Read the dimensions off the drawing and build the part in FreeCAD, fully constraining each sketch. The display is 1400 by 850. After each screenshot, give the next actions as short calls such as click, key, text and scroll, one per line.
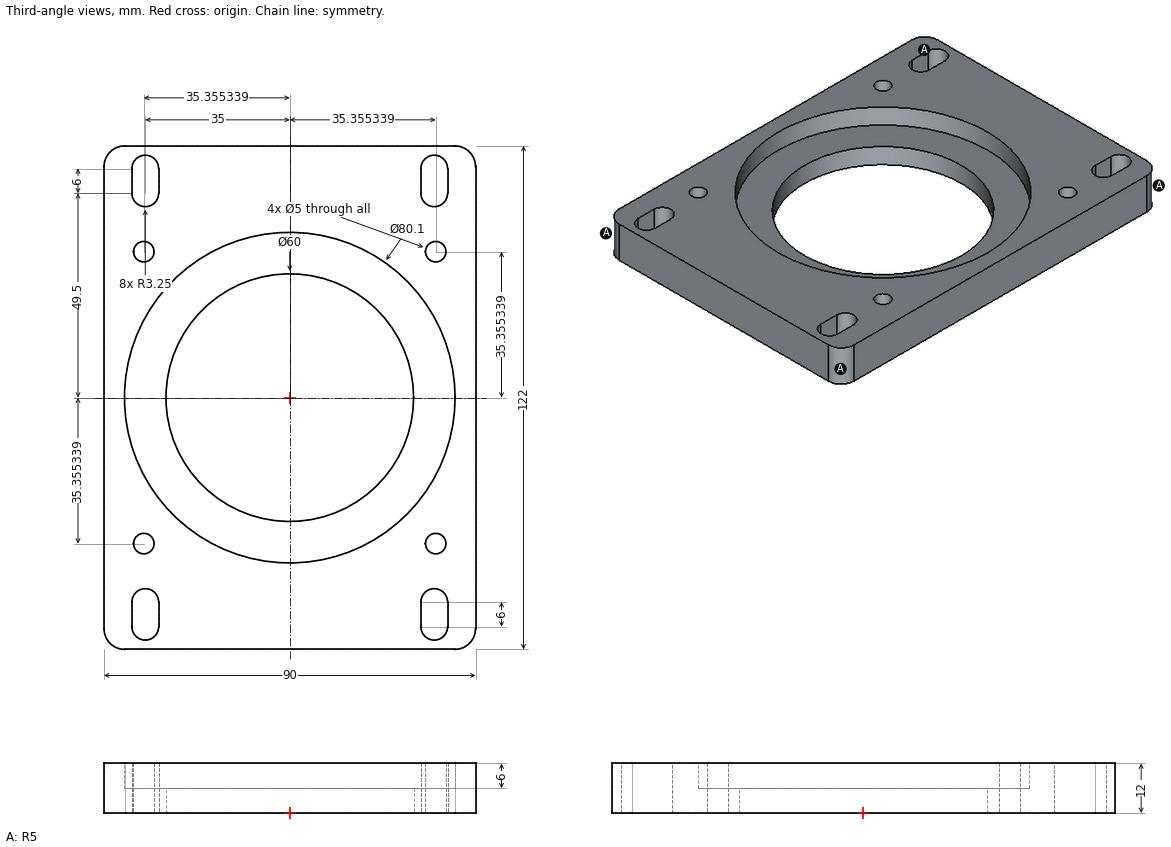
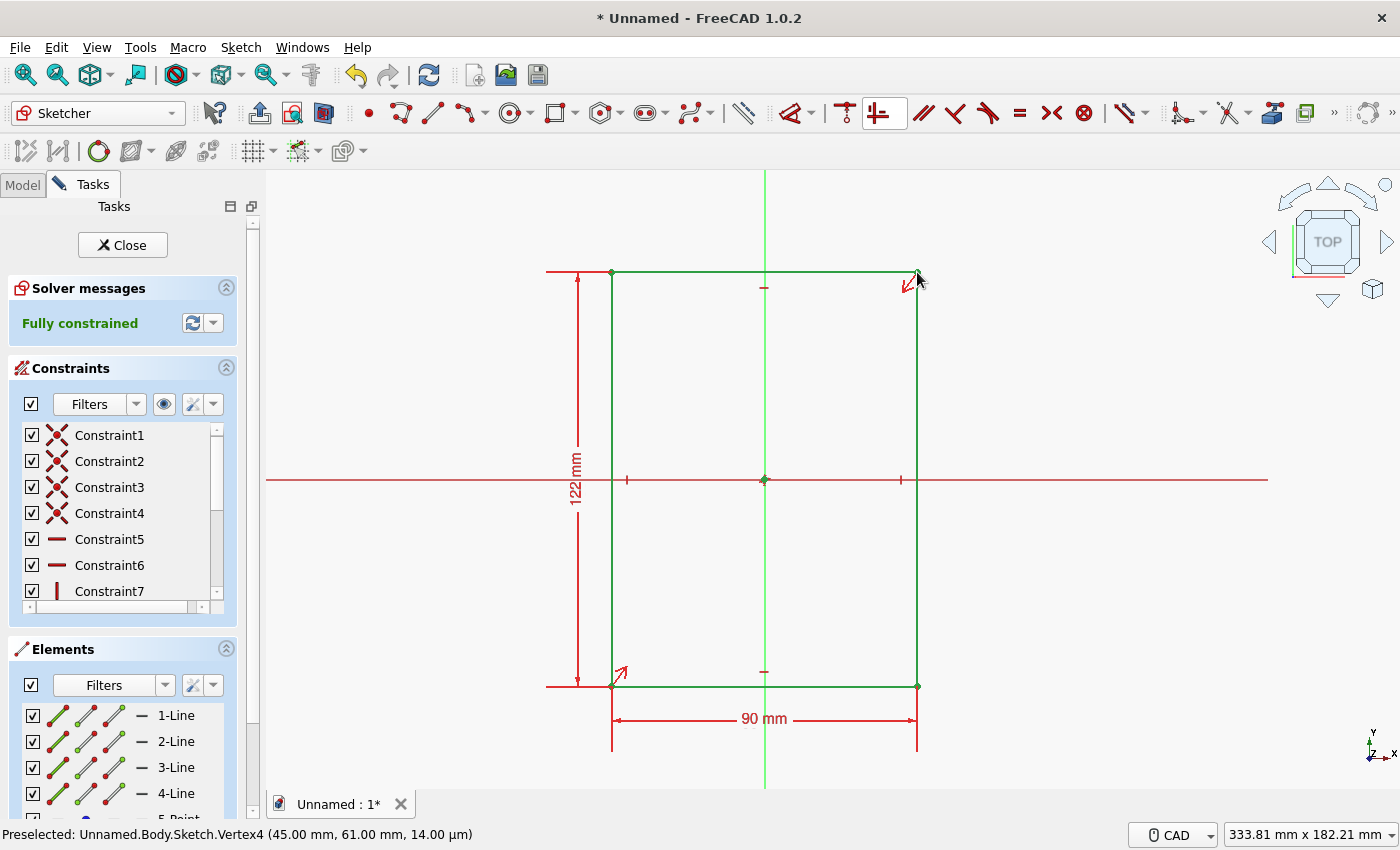
click(123, 245)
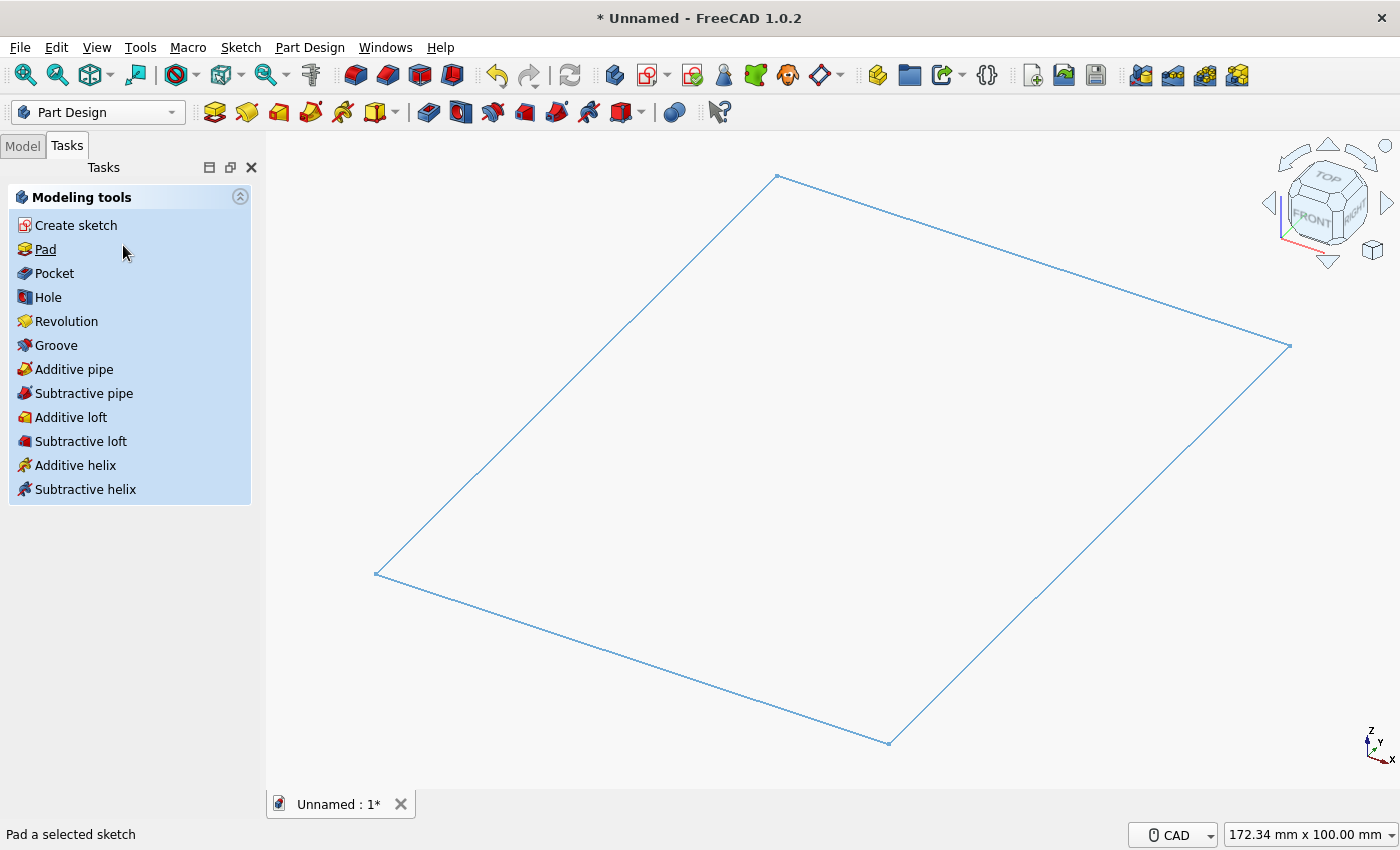
click(216, 112)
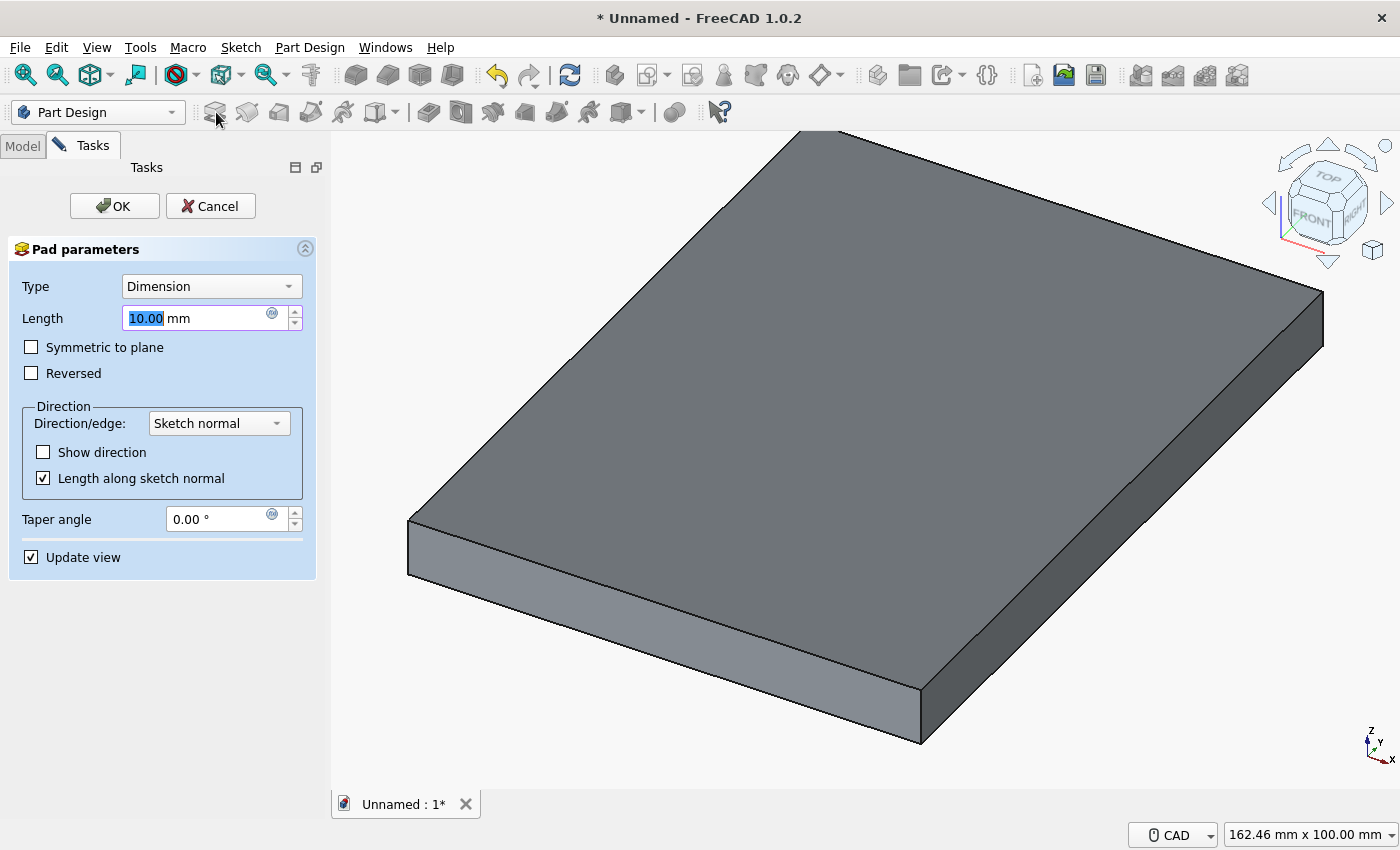
text(12)
key(Tab)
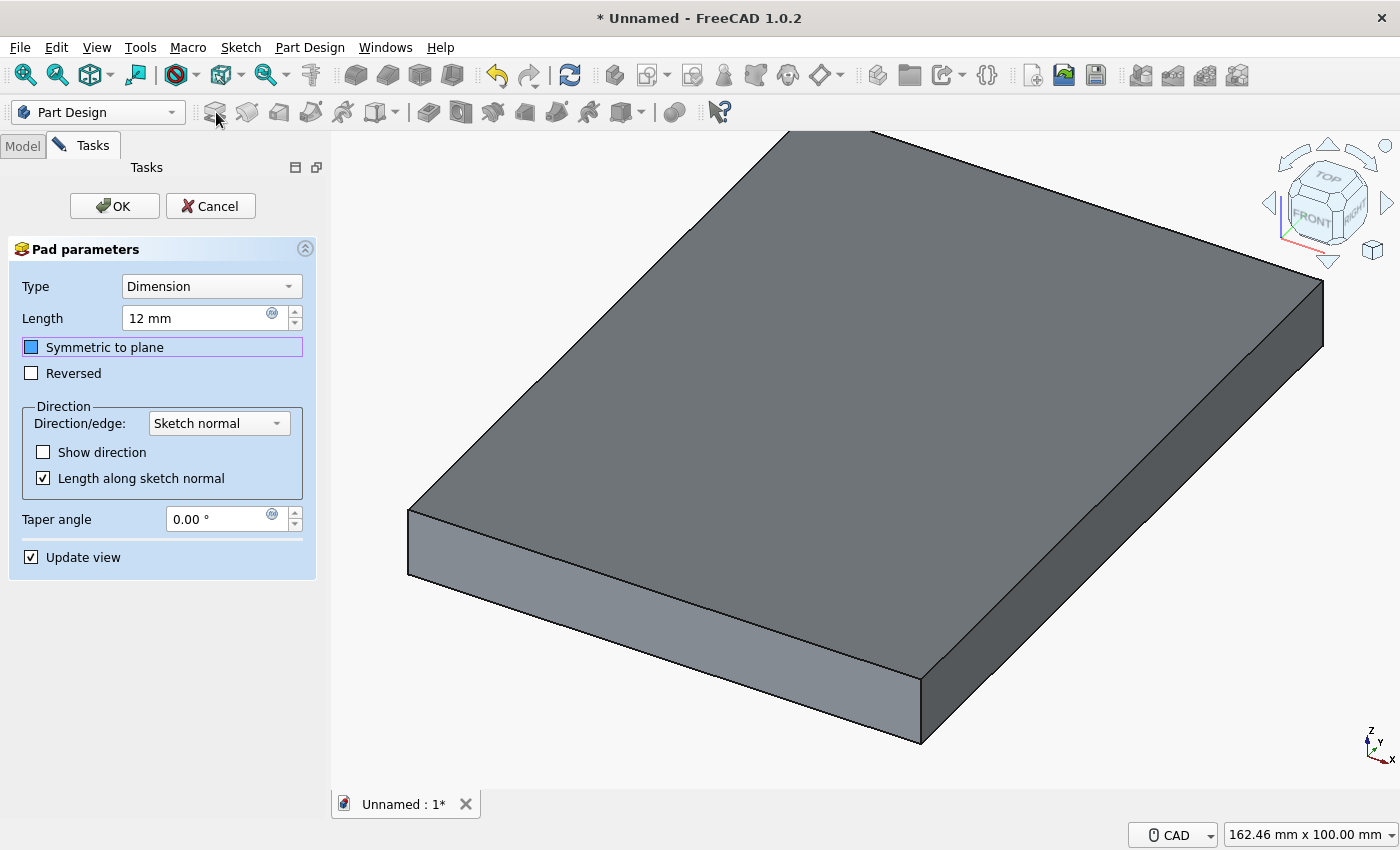
click(115, 206)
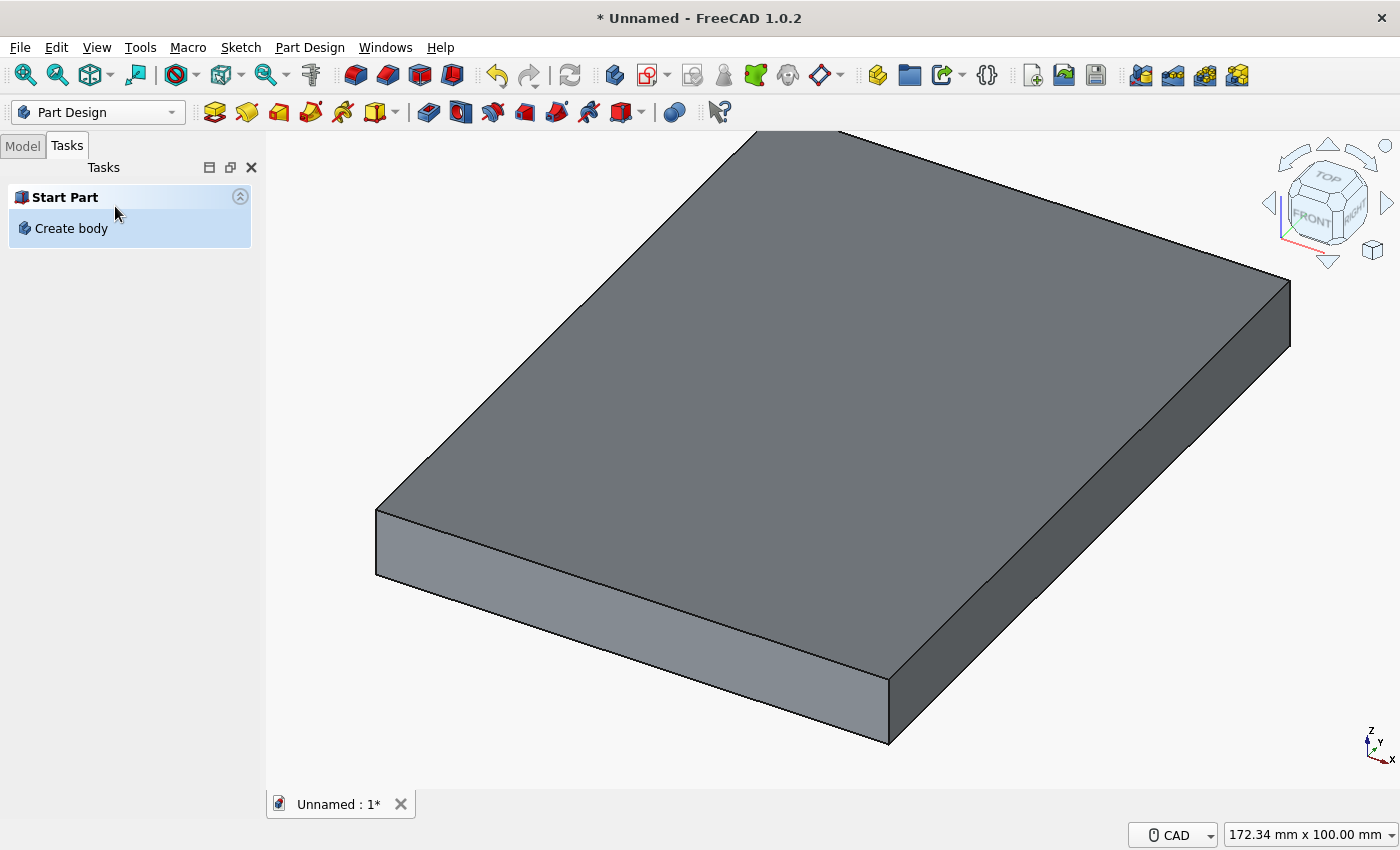
click(26, 76)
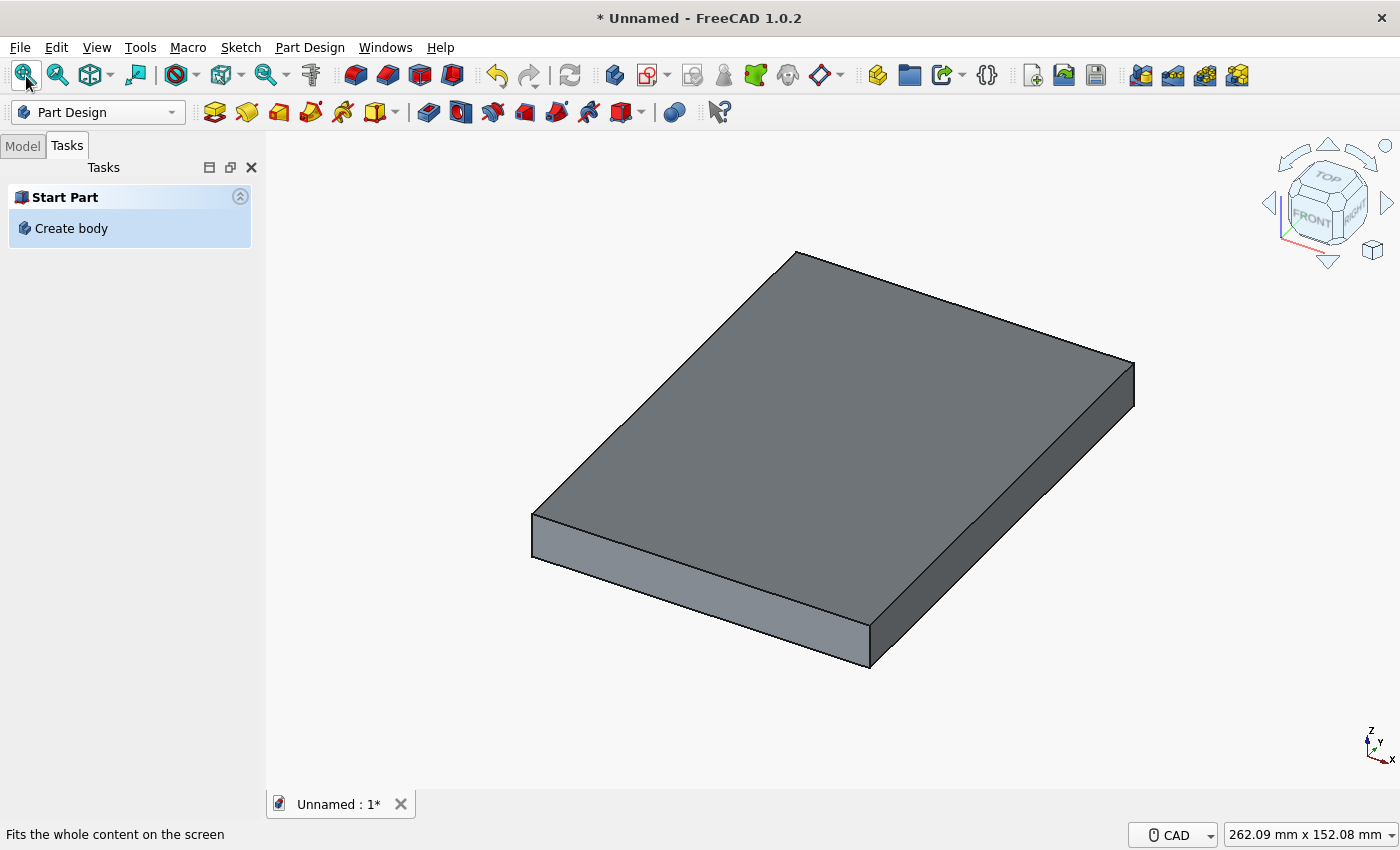
click(833, 438)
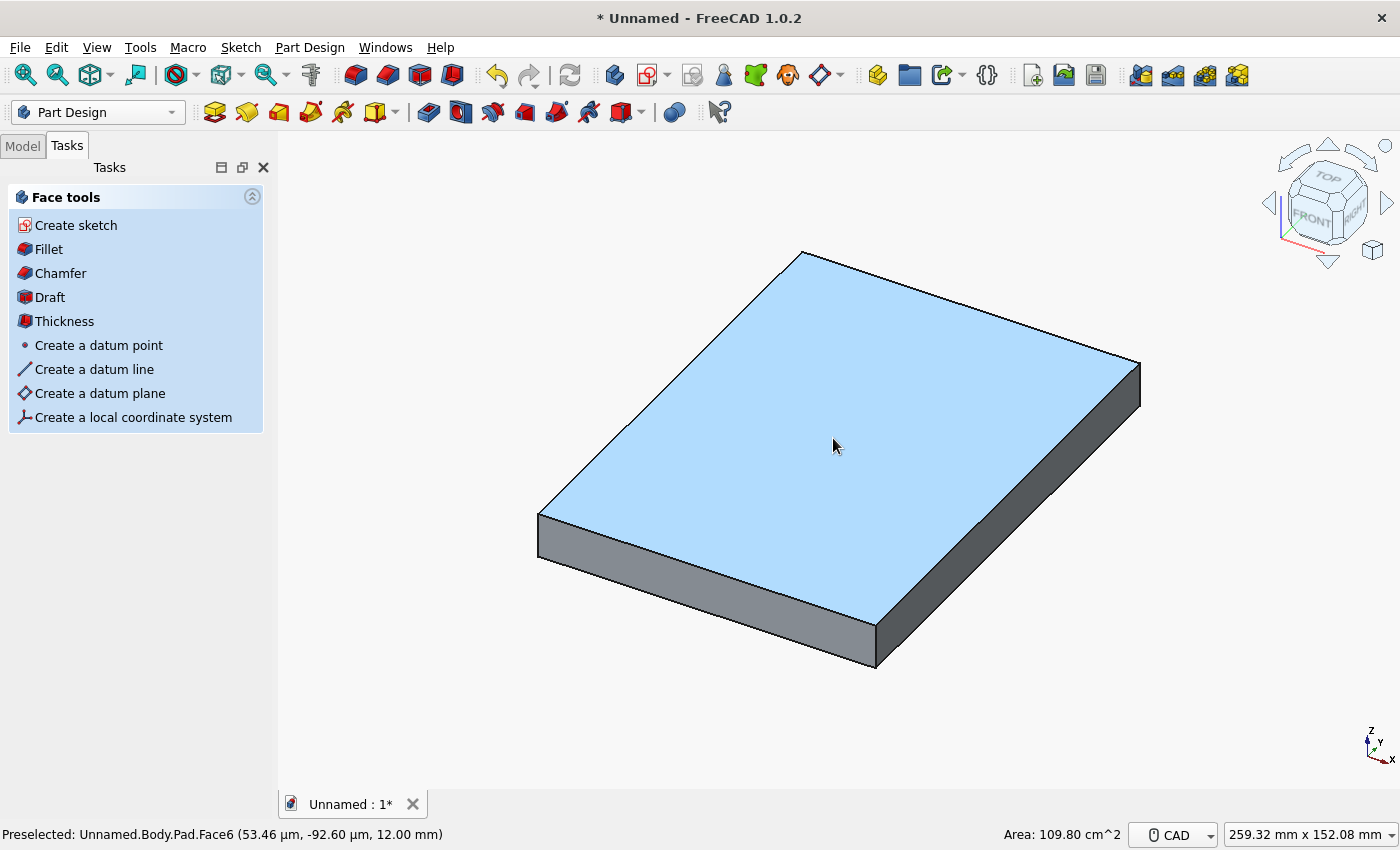
click(648, 76)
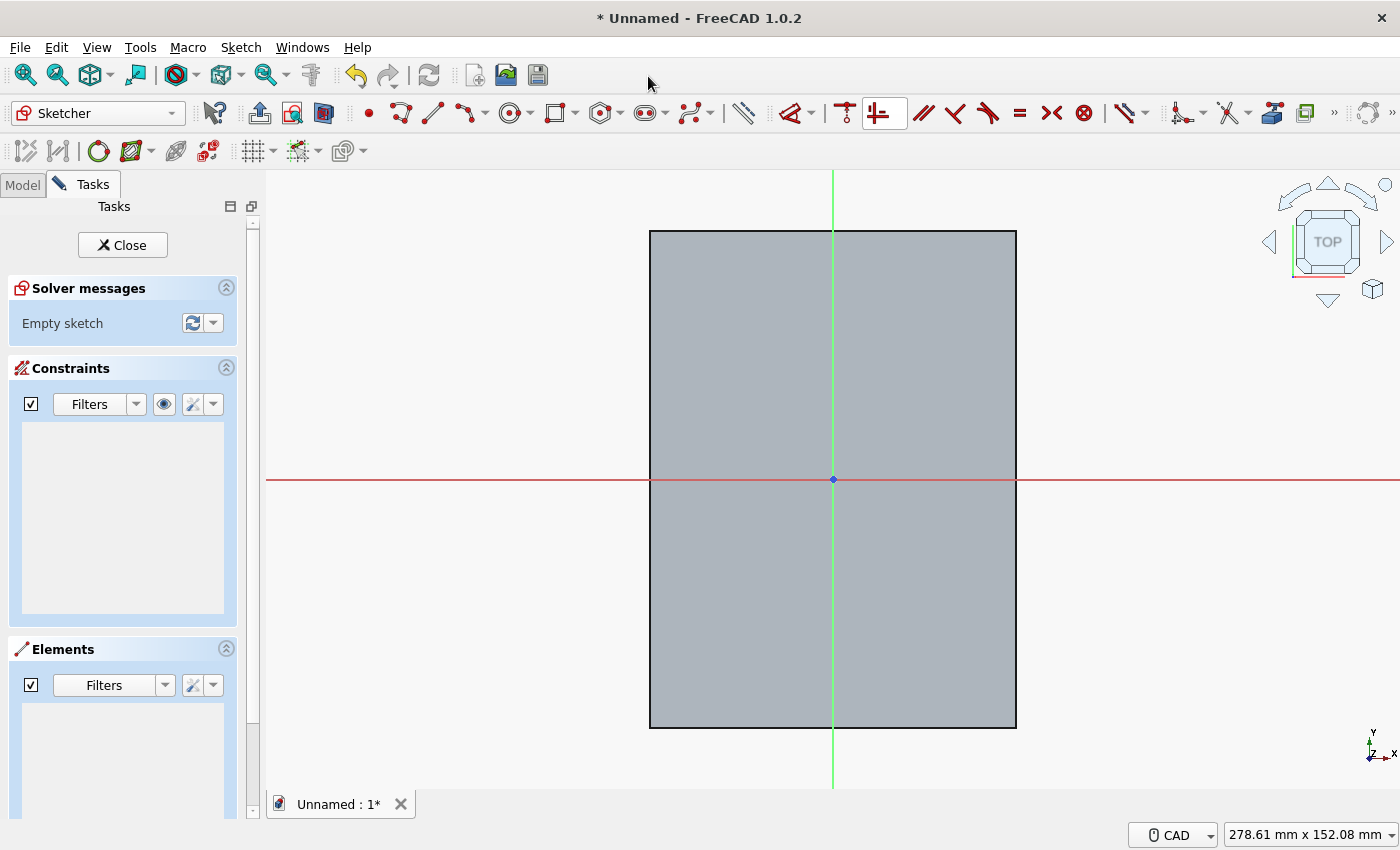
scroll(972, 480, up, 2)